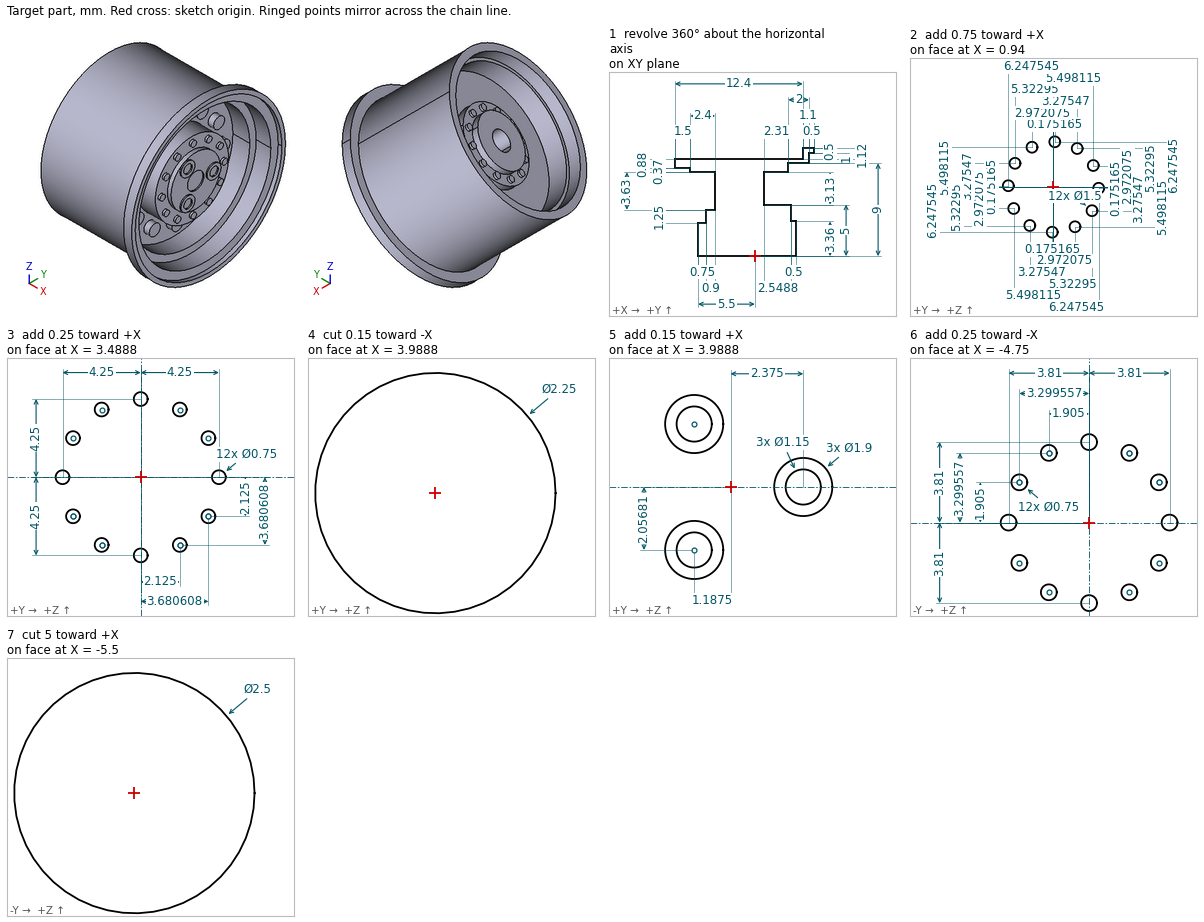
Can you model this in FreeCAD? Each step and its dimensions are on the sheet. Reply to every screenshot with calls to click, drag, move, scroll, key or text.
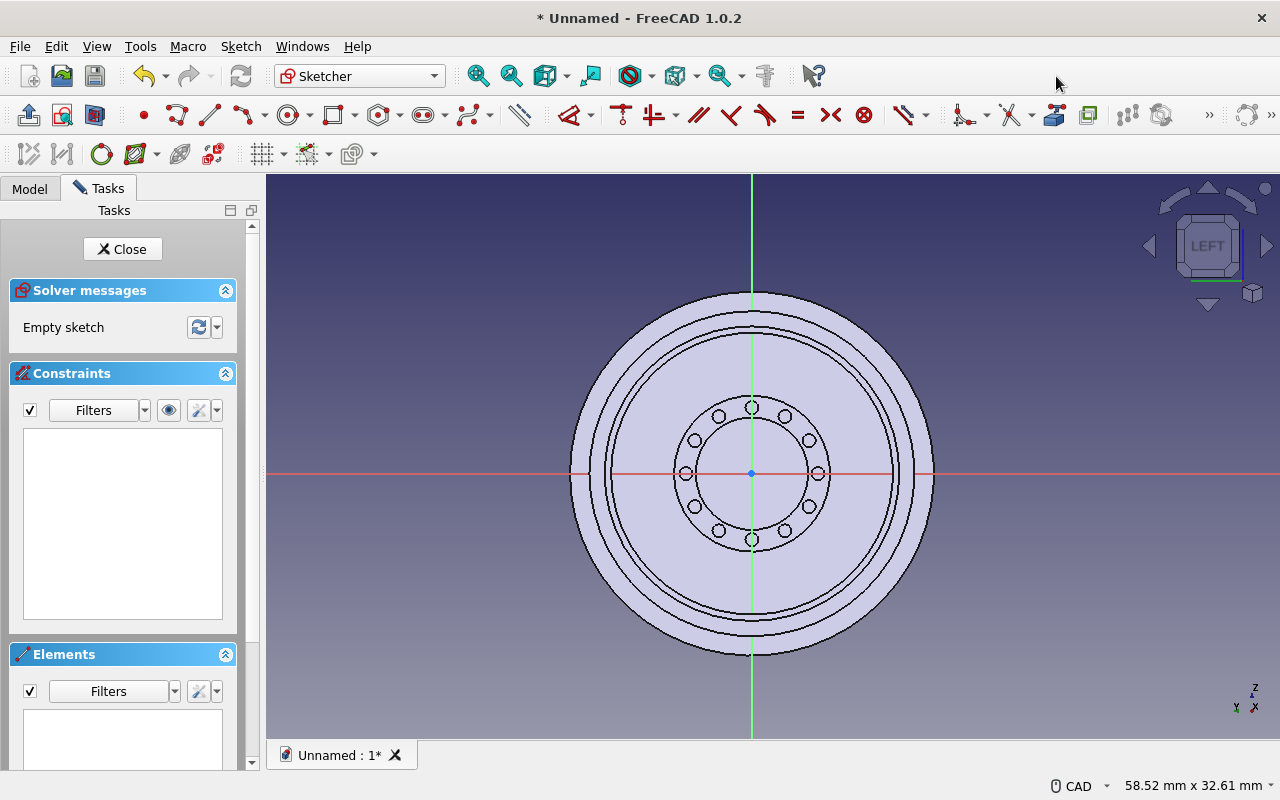
scroll(758, 476, up, 11)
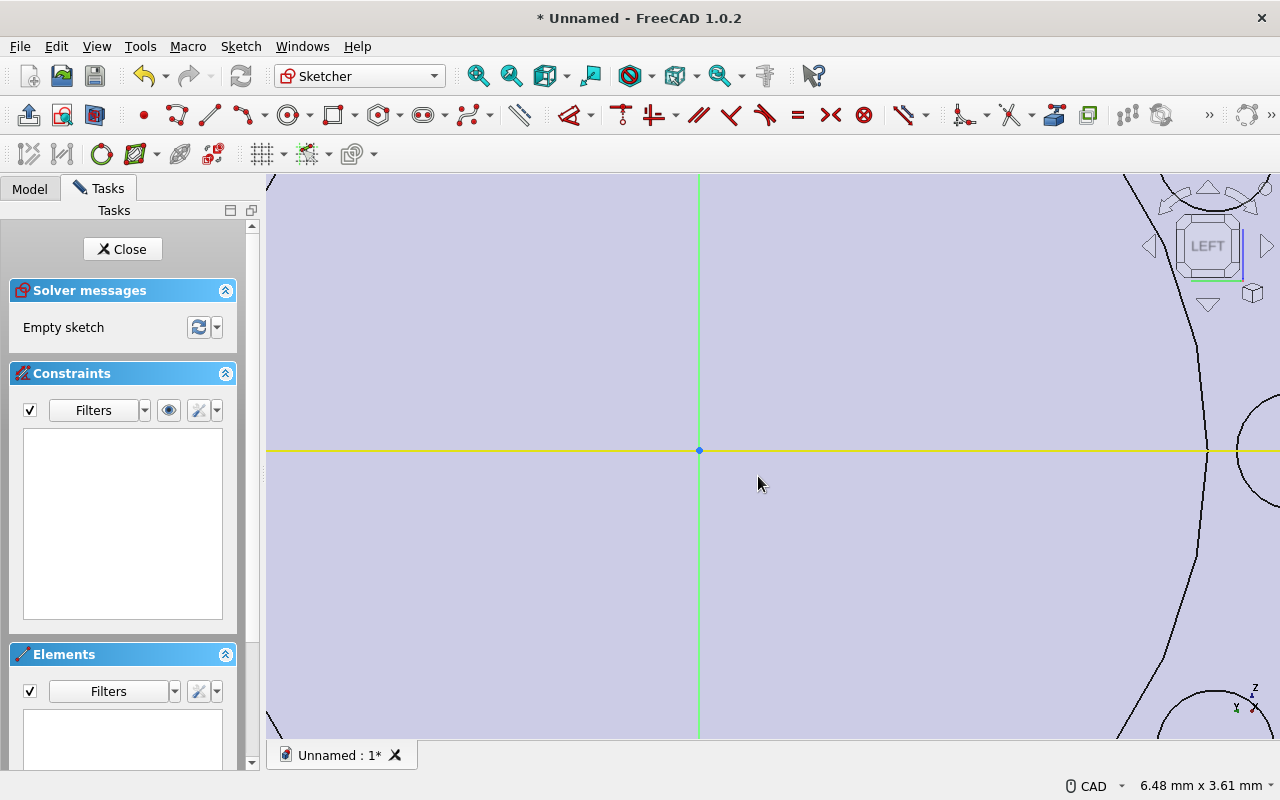
click(288, 116)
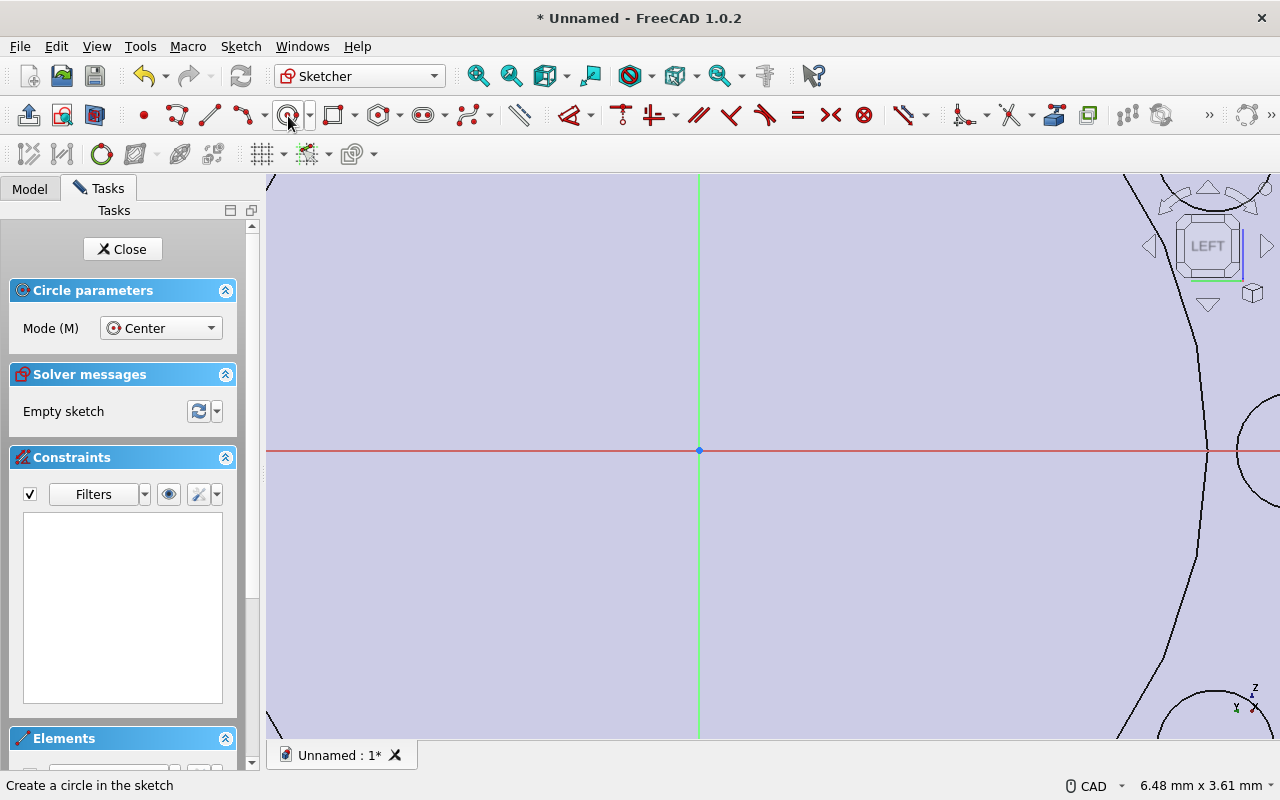
click(699, 451)
move(838, 313)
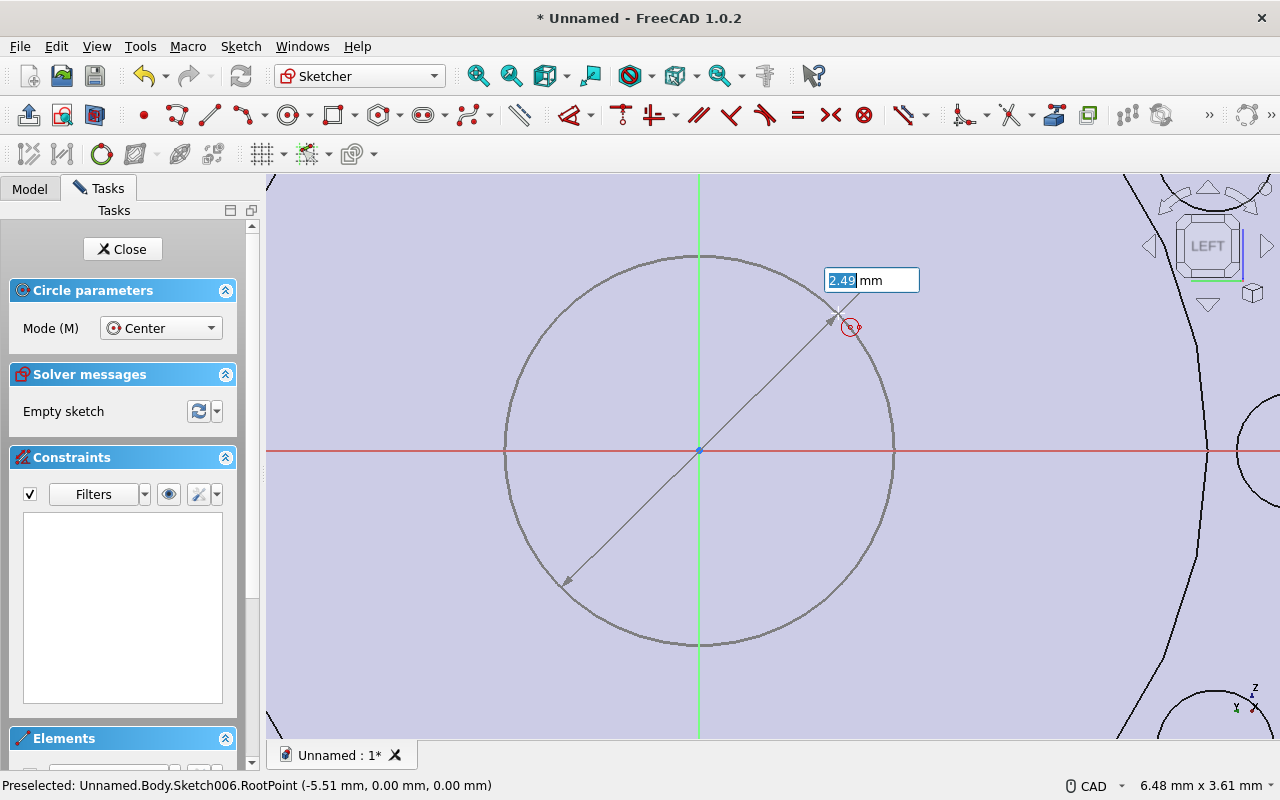
text(2.5)
key(Return)
key(Escape)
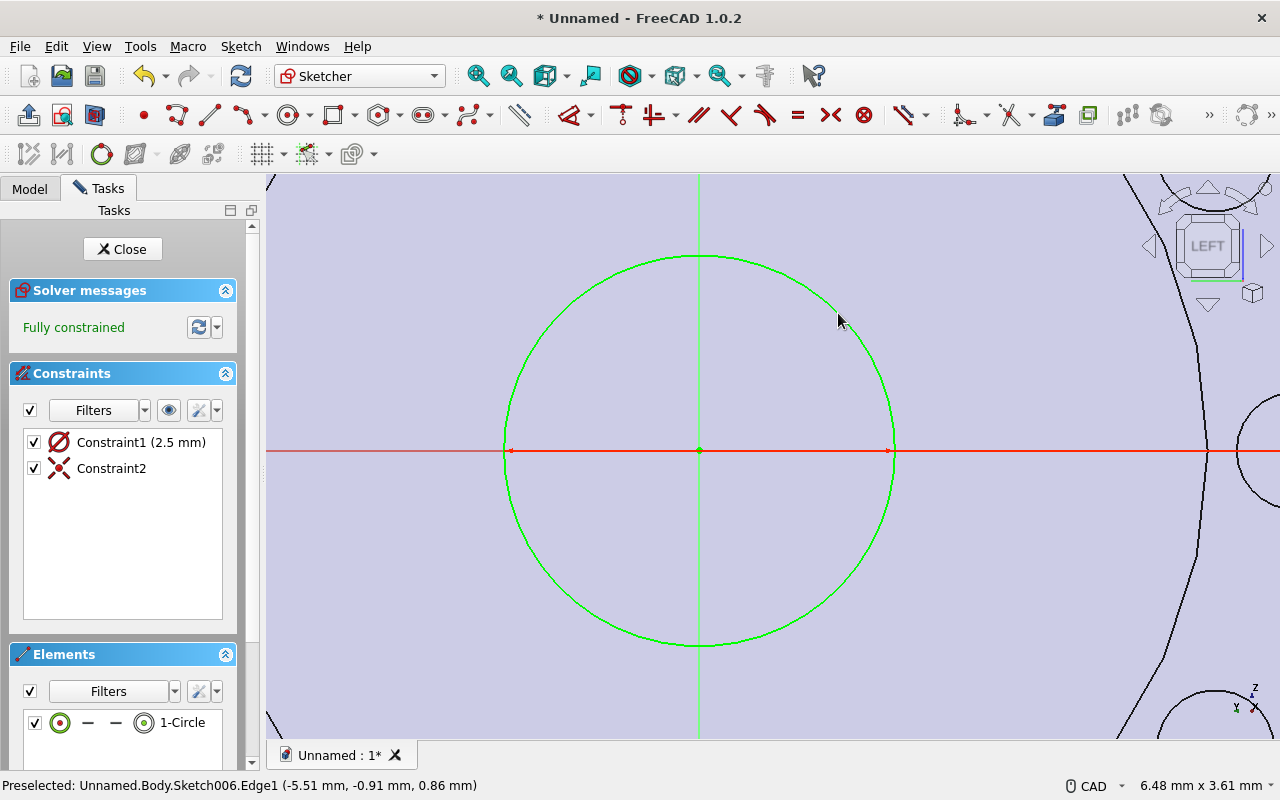
click(123, 249)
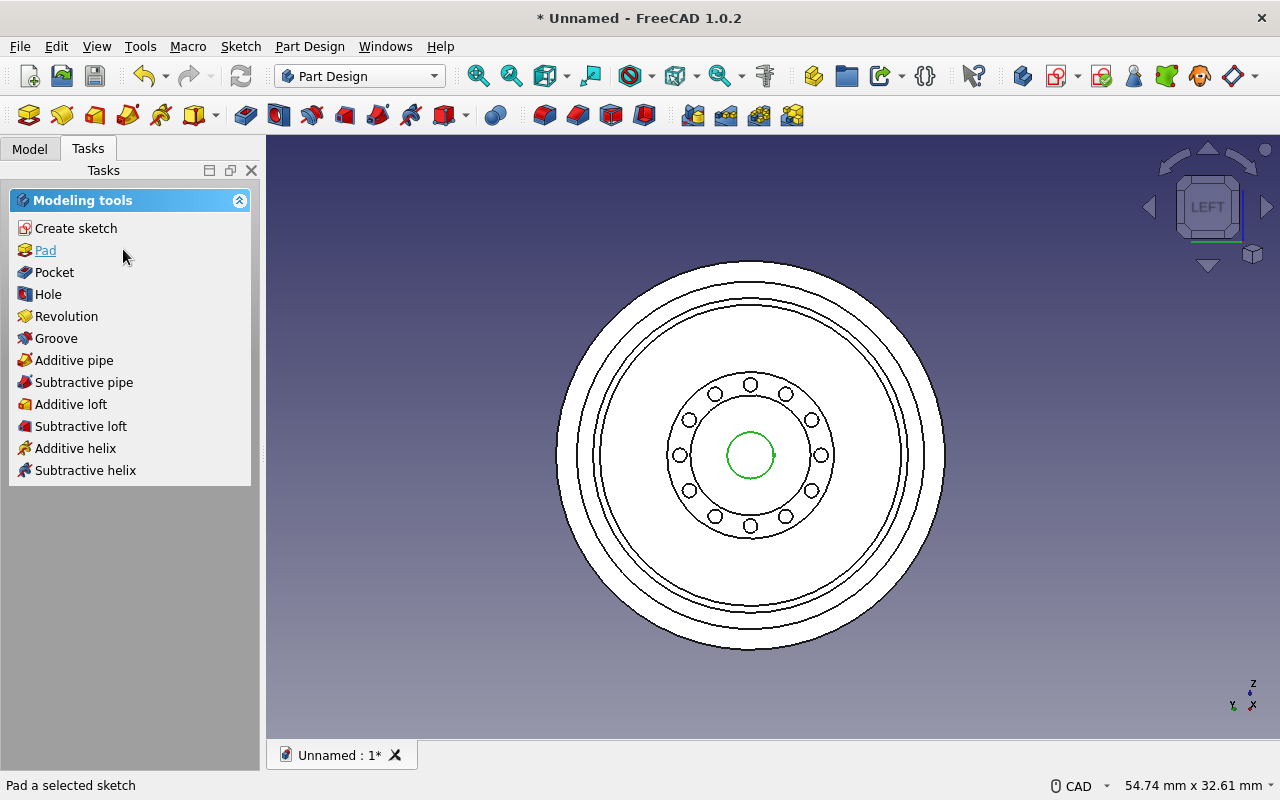
click(246, 116)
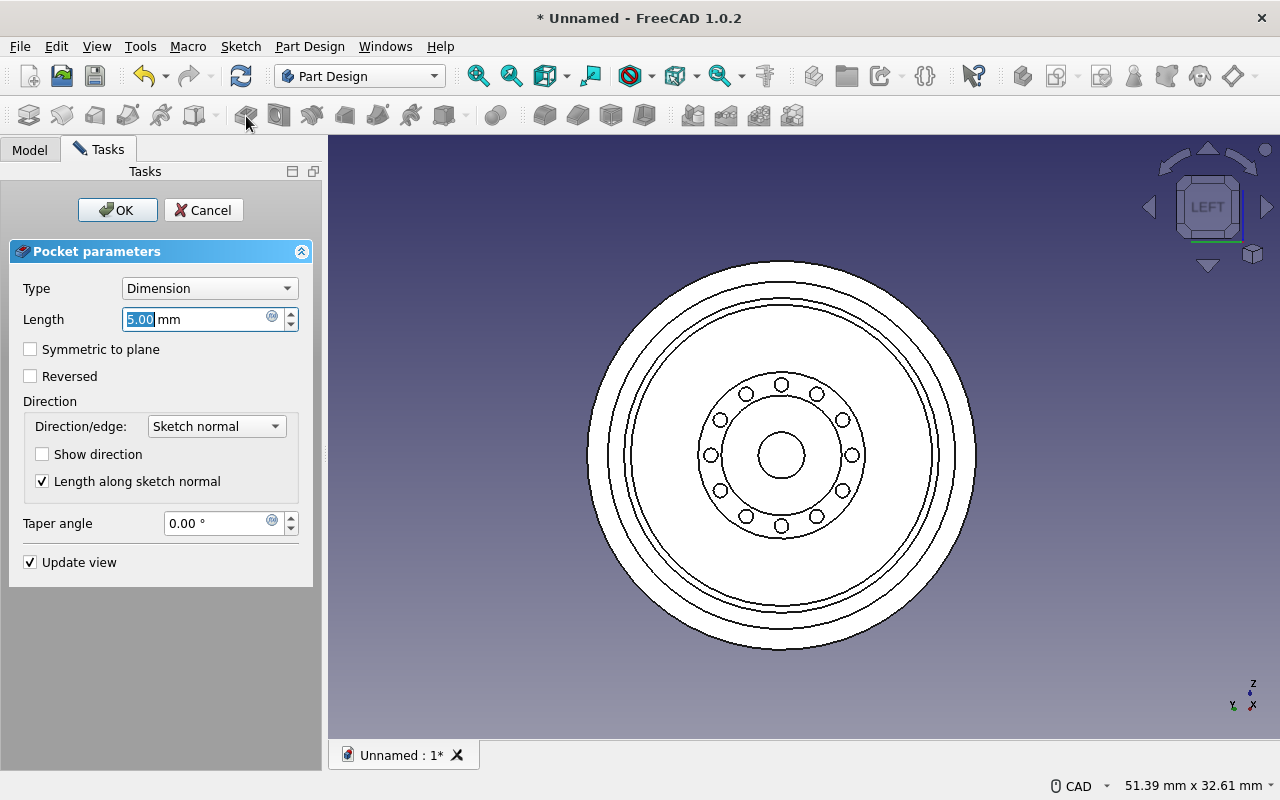
text(5)
key(Tab)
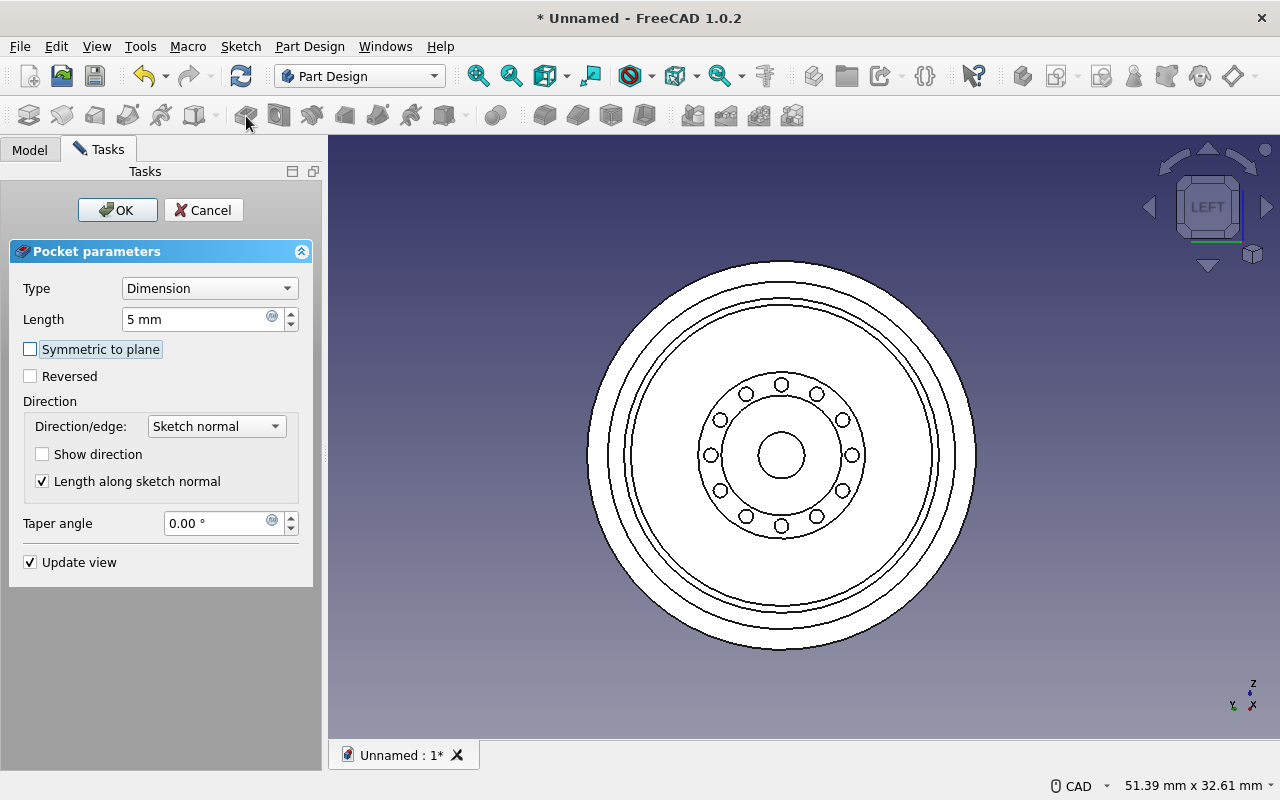
click(118, 210)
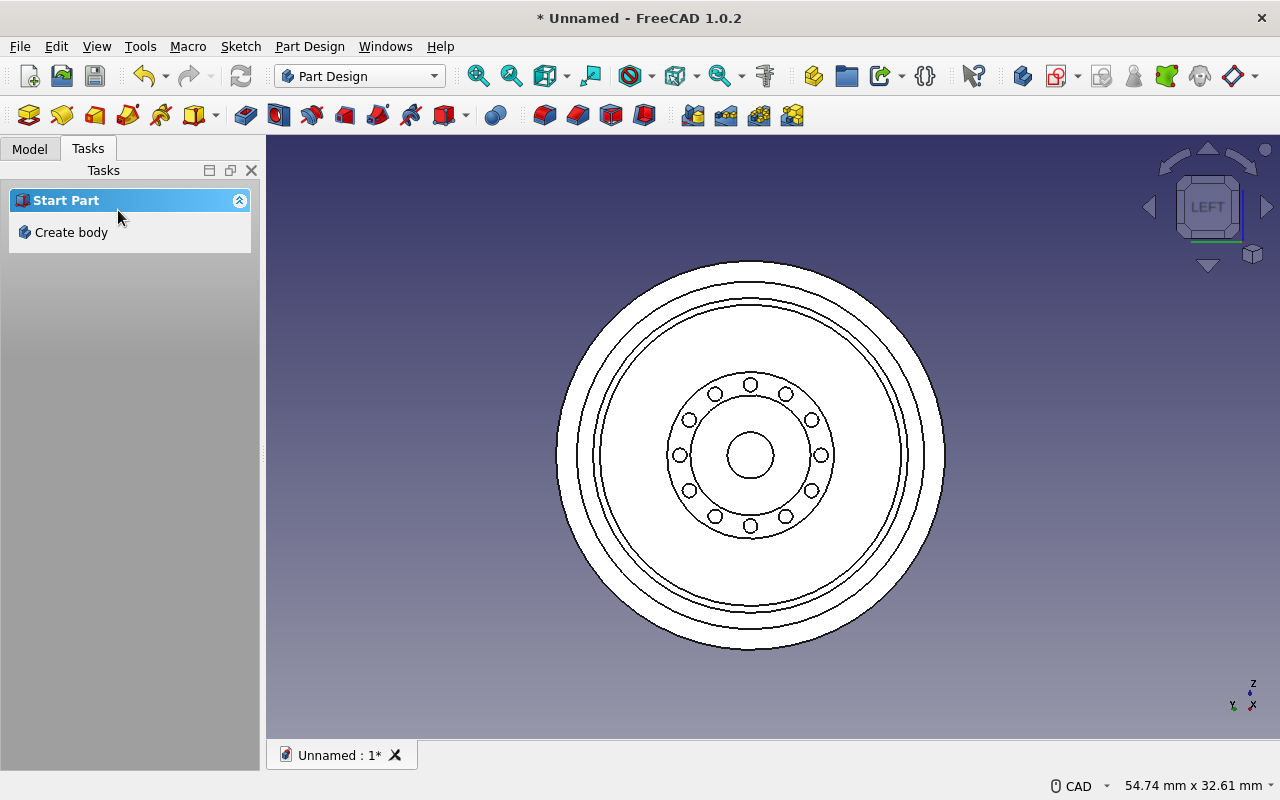
key(0)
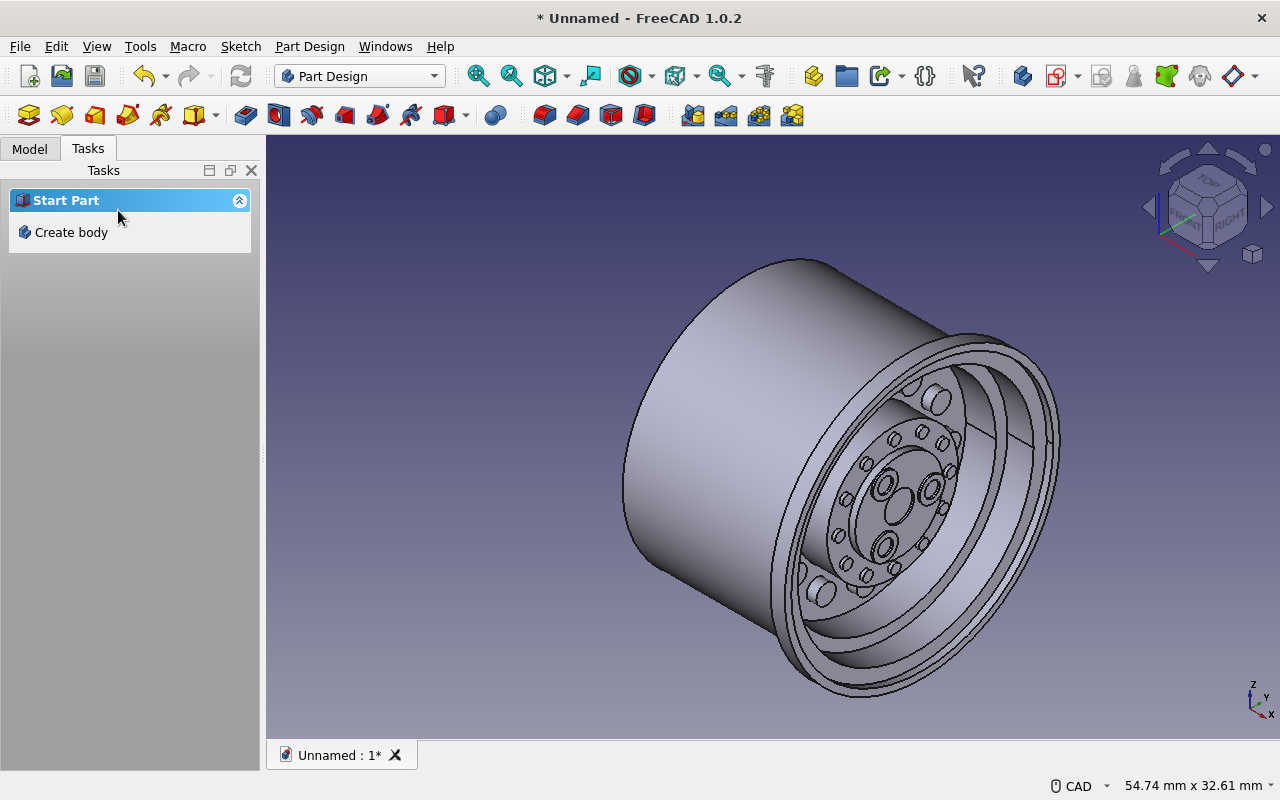
click(479, 76)